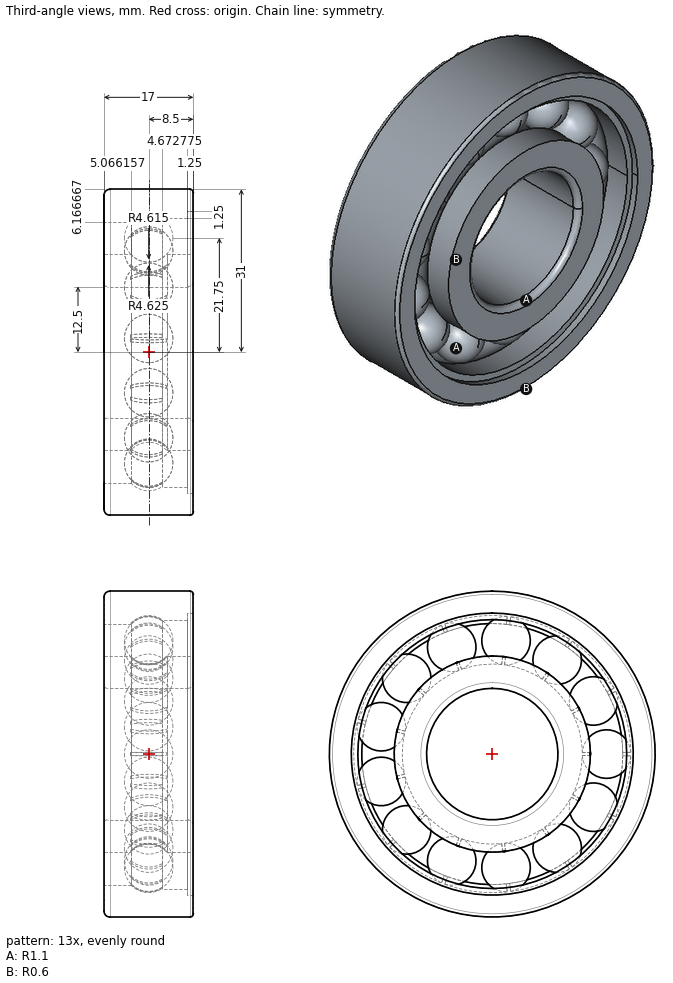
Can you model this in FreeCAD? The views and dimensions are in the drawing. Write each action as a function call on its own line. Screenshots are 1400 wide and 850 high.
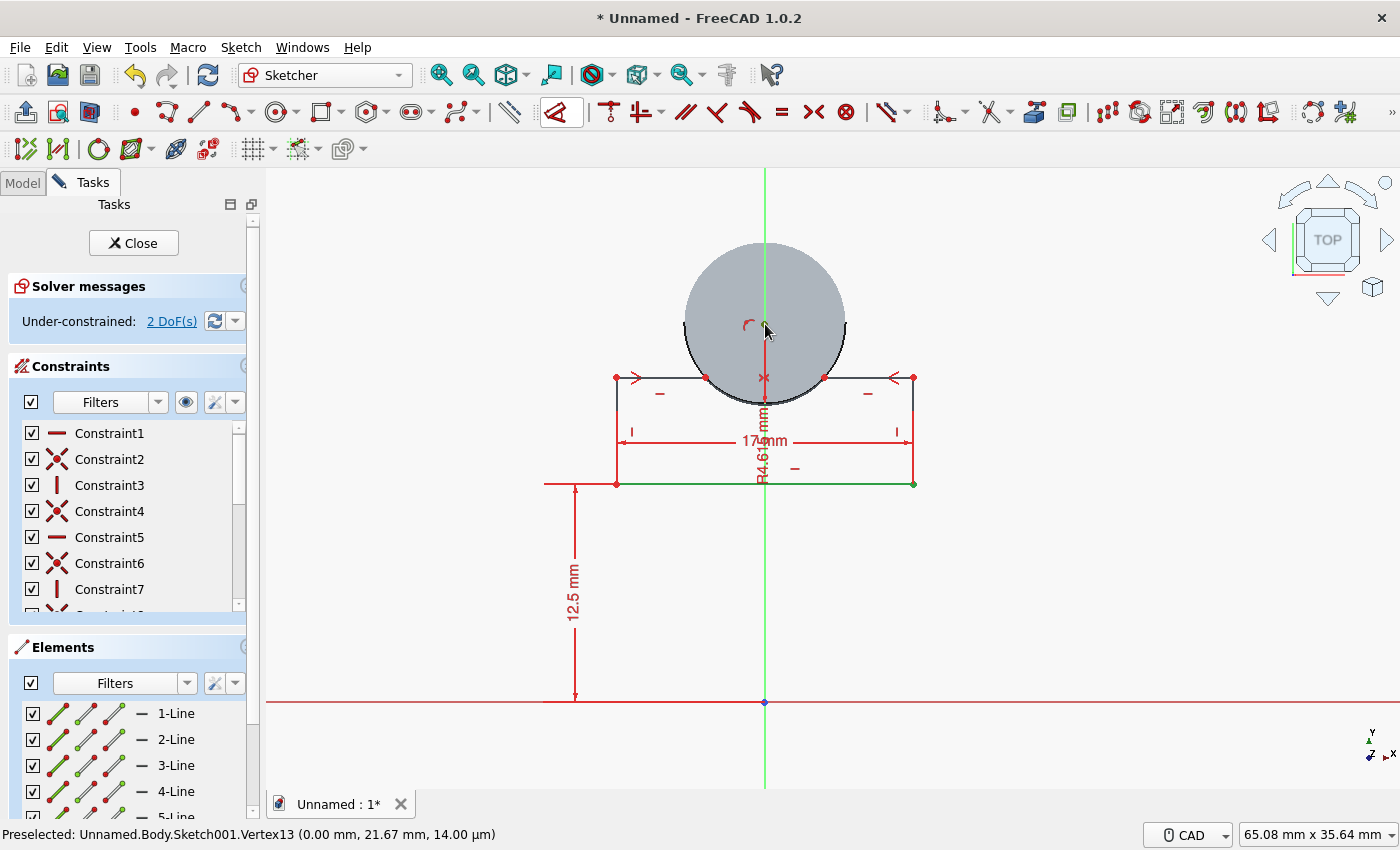
key(i)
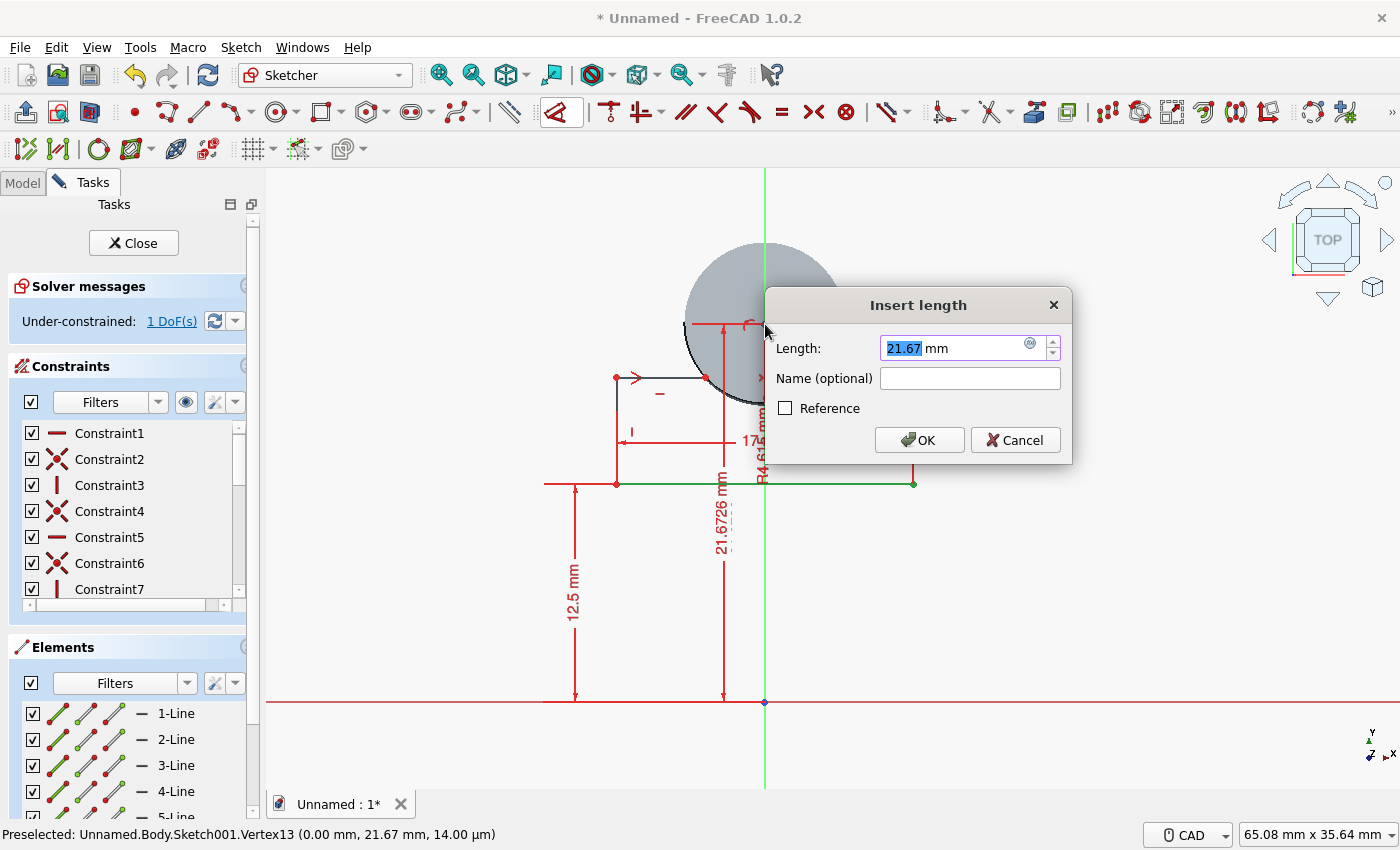
text(21.75)
key(Return)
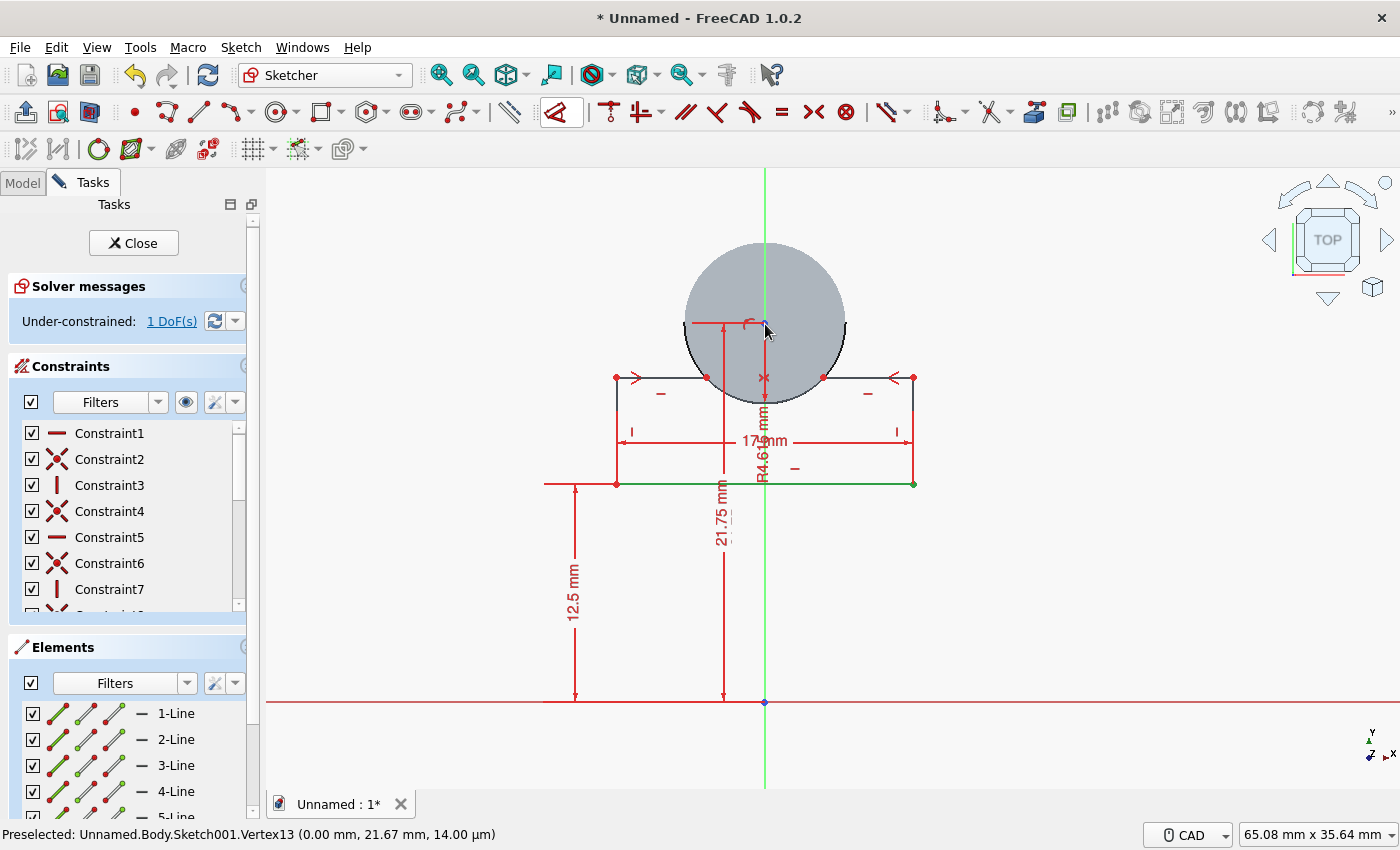
click(679, 378)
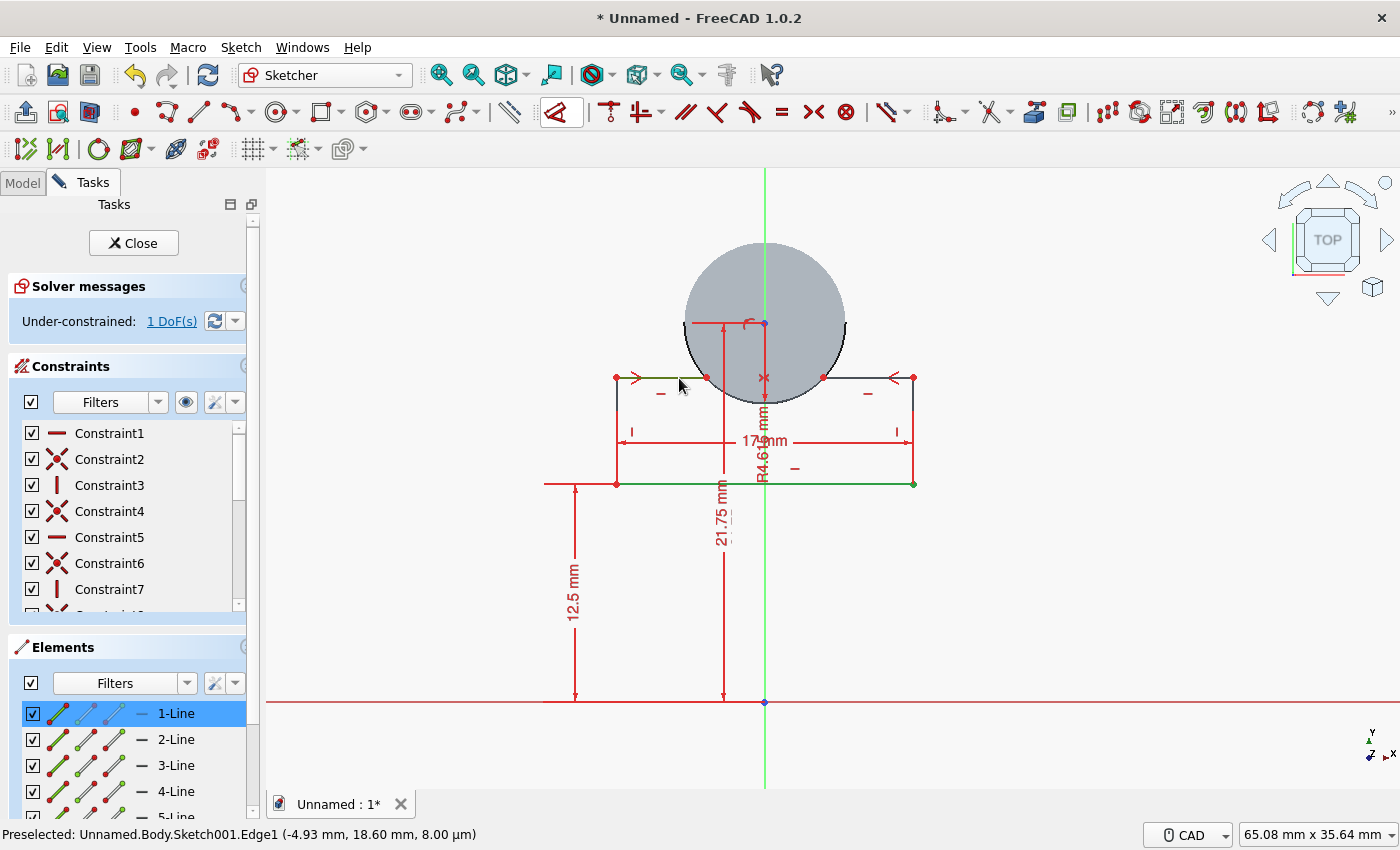
click(578, 112)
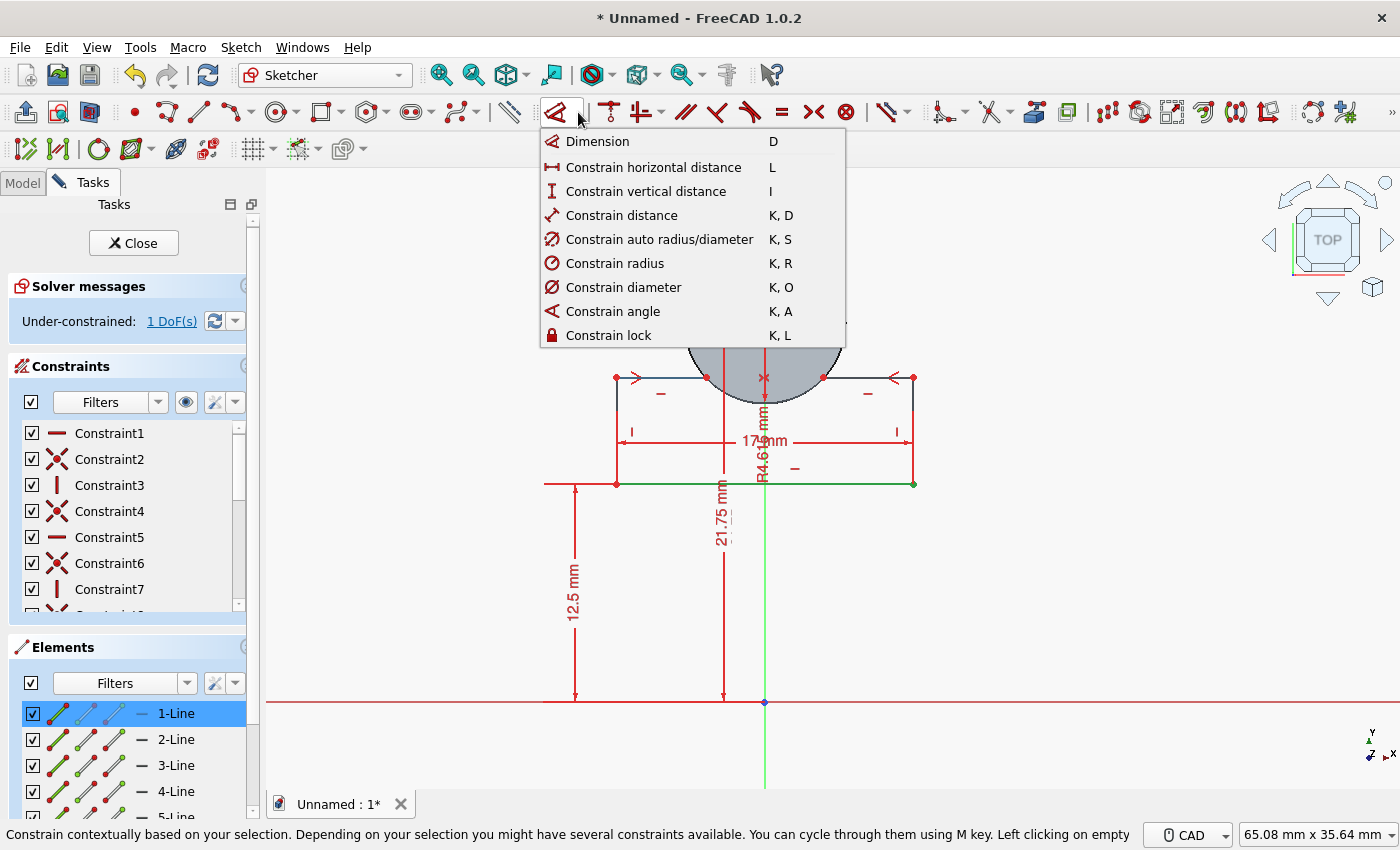
click(693, 167)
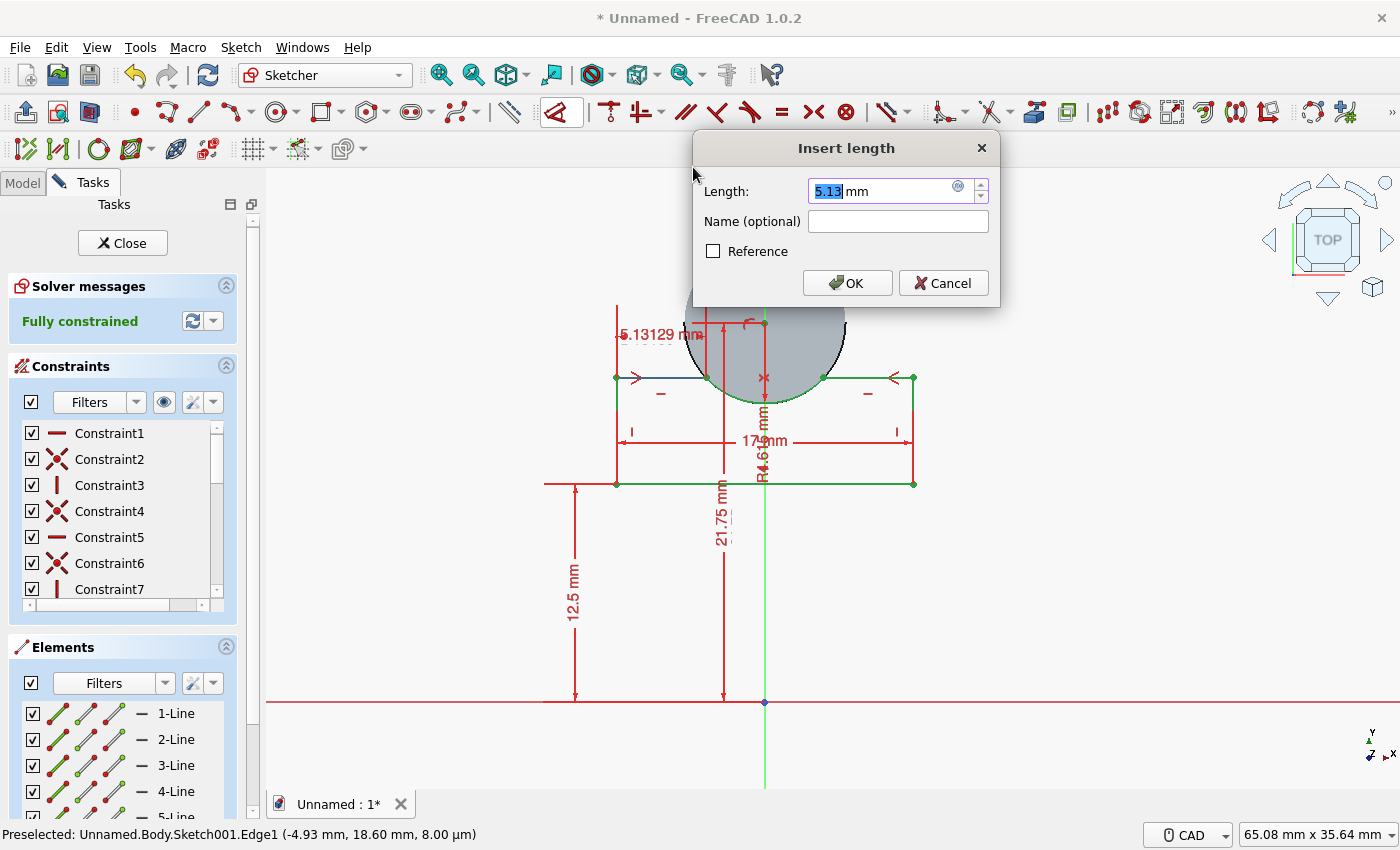
text(5.066157)
key(Return)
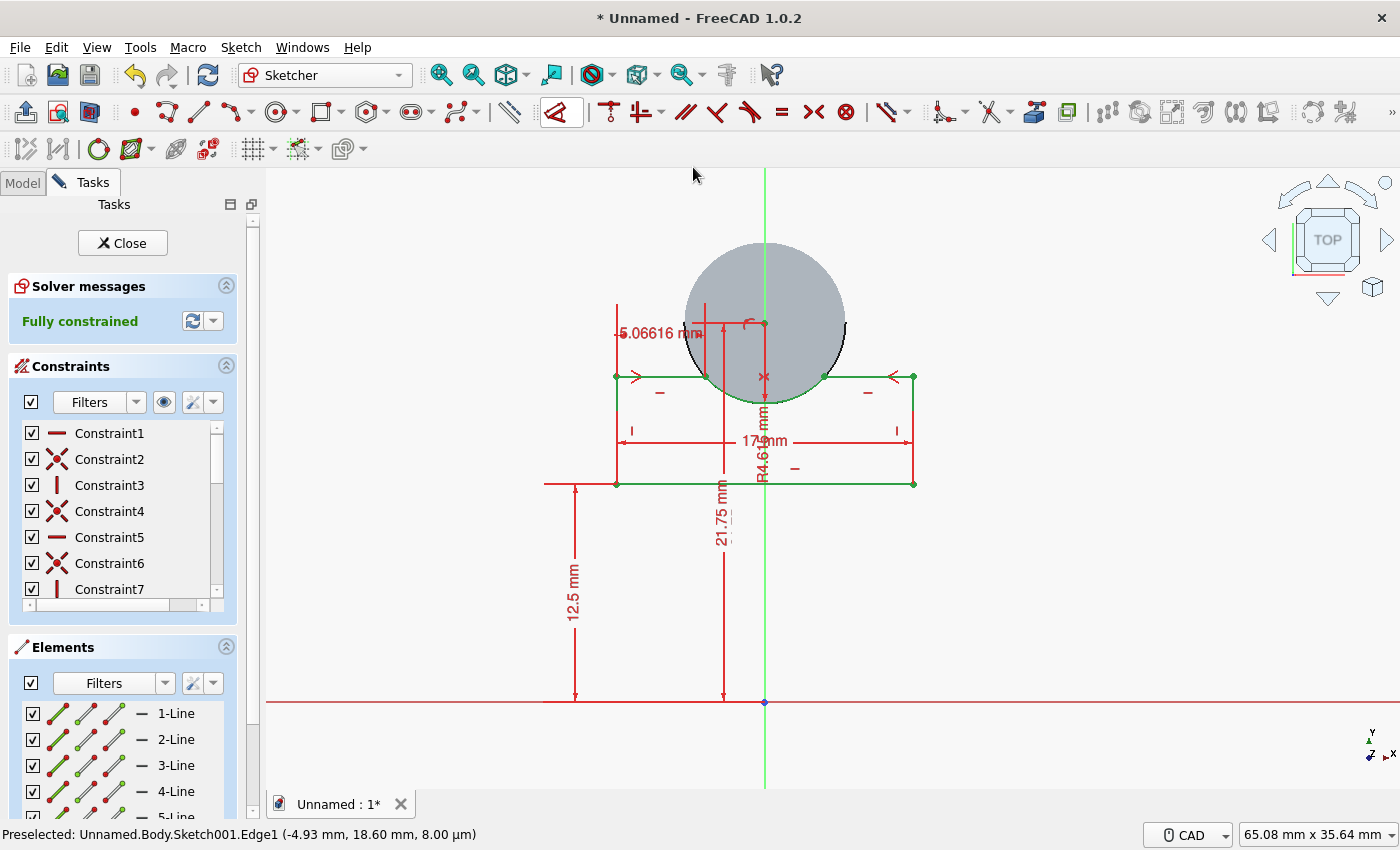
click(123, 243)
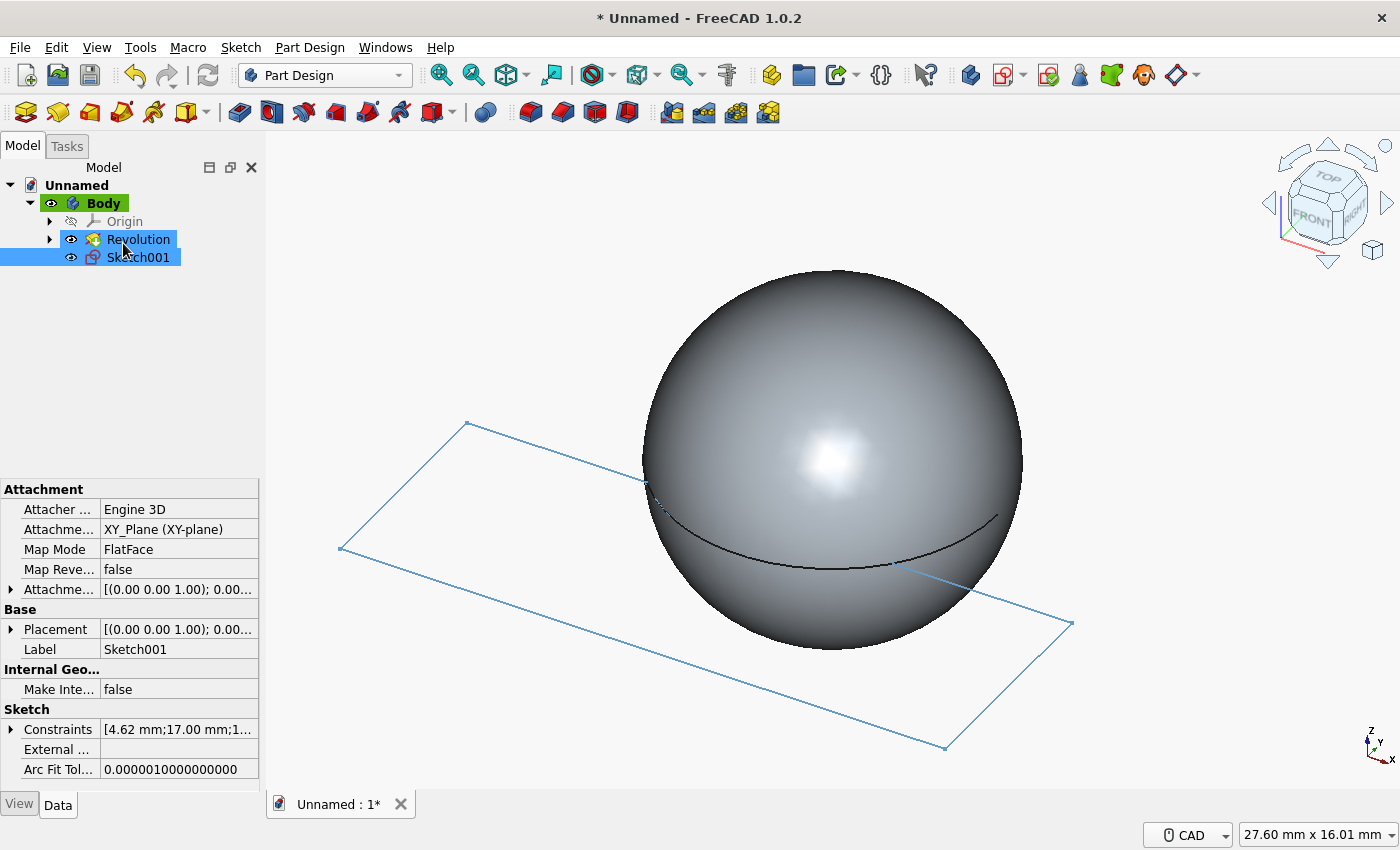
click(58, 112)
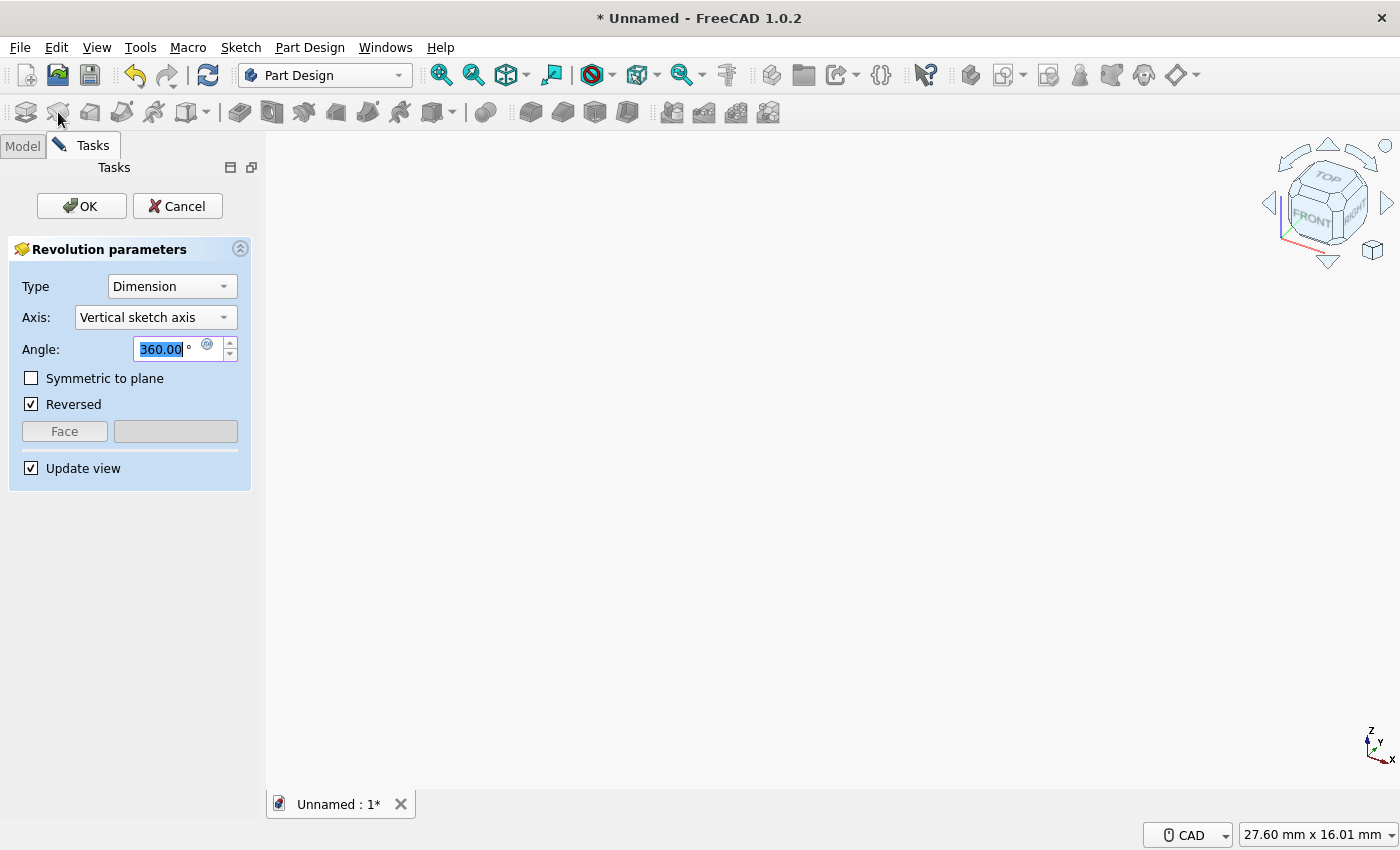
click(156, 318)